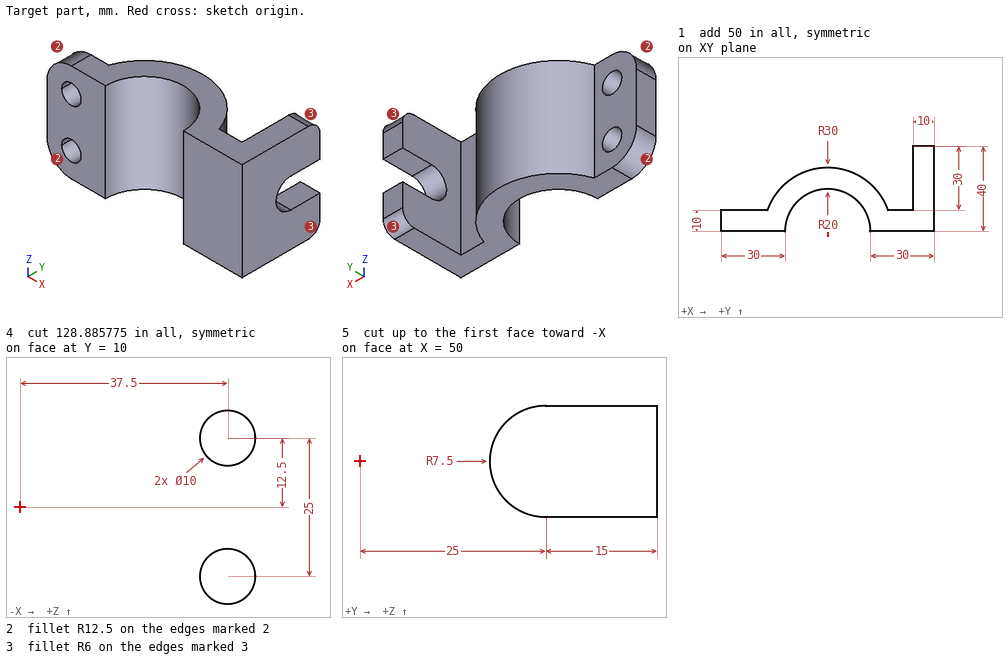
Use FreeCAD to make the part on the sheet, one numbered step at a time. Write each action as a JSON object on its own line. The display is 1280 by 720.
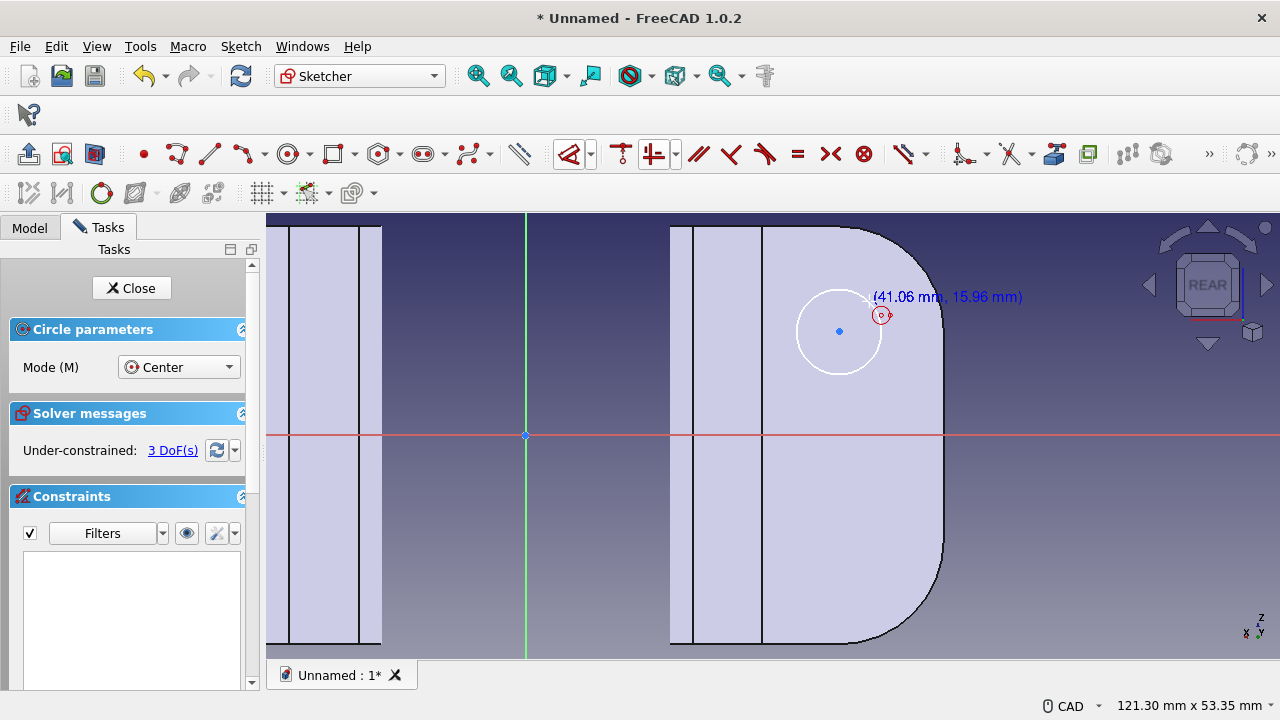
{"action": "left_click", "coordinate": [839, 540]}
{"action": "left_click", "coordinate": [869, 510]}
{"action": "key", "text": "Escape"}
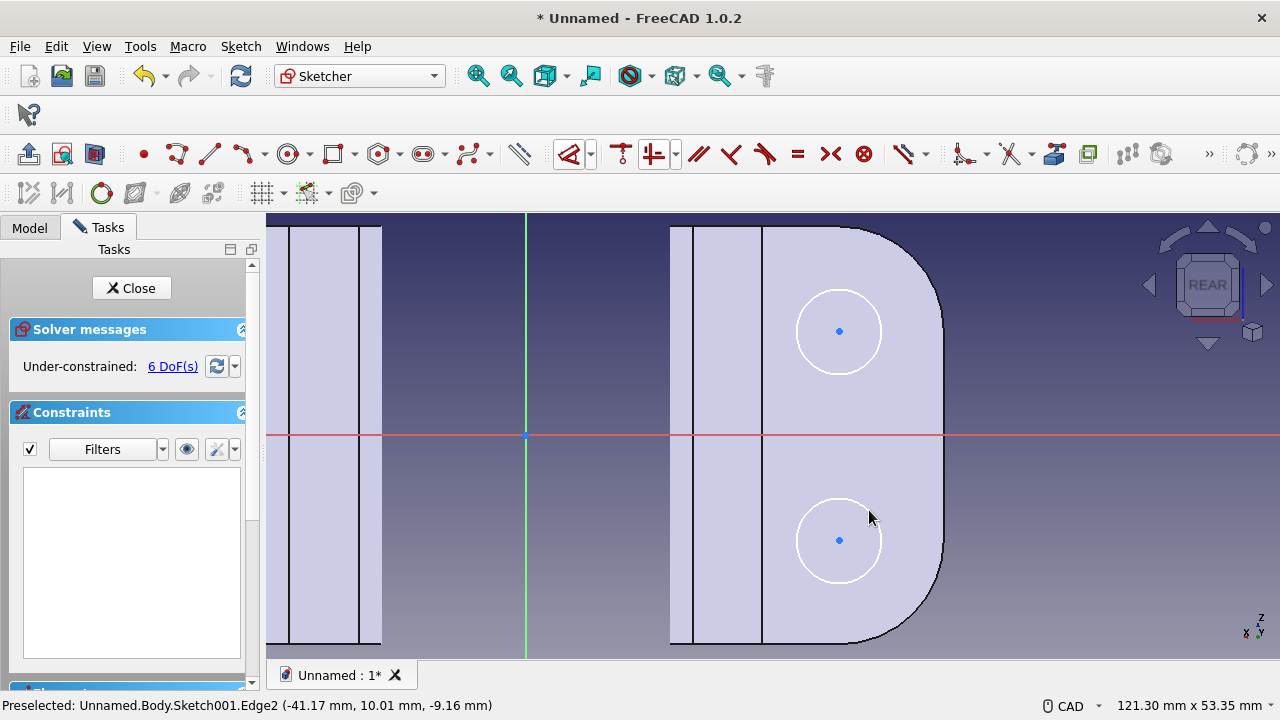
{"action": "left_click", "coordinate": [869, 302]}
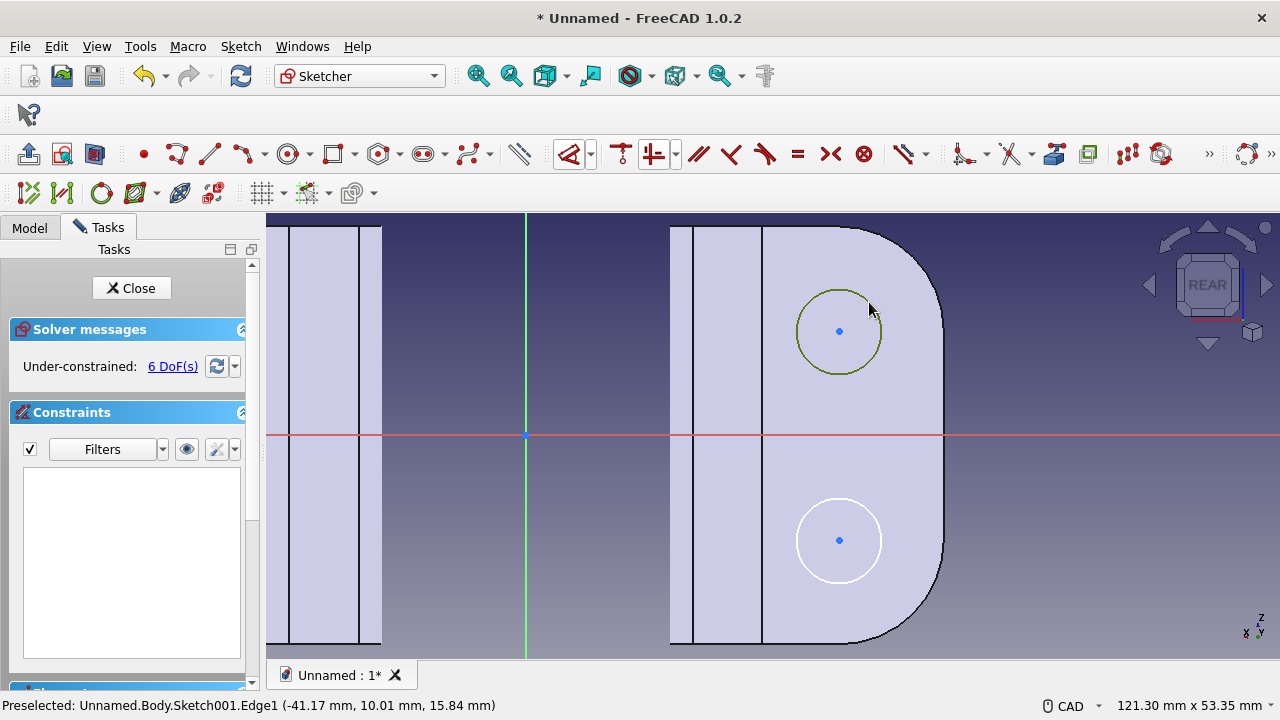
{"action": "left_click", "coordinate": [869, 511]}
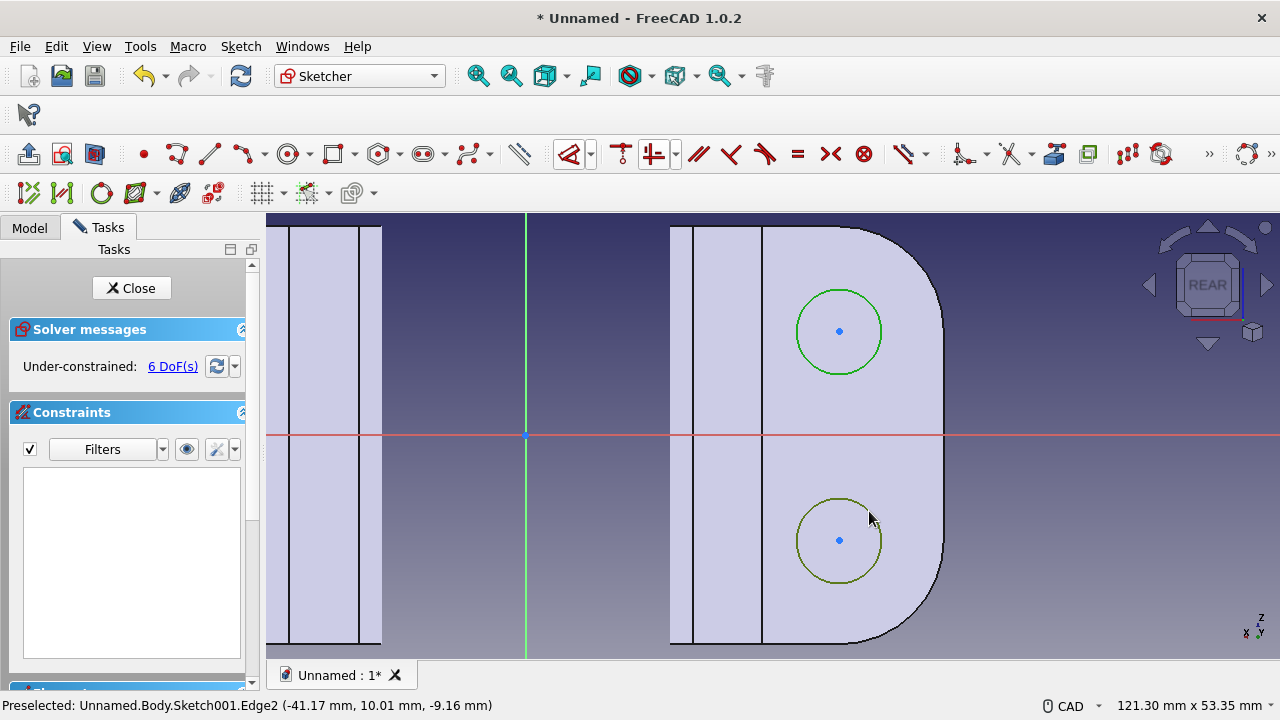
{"action": "left_click", "coordinate": [798, 154]}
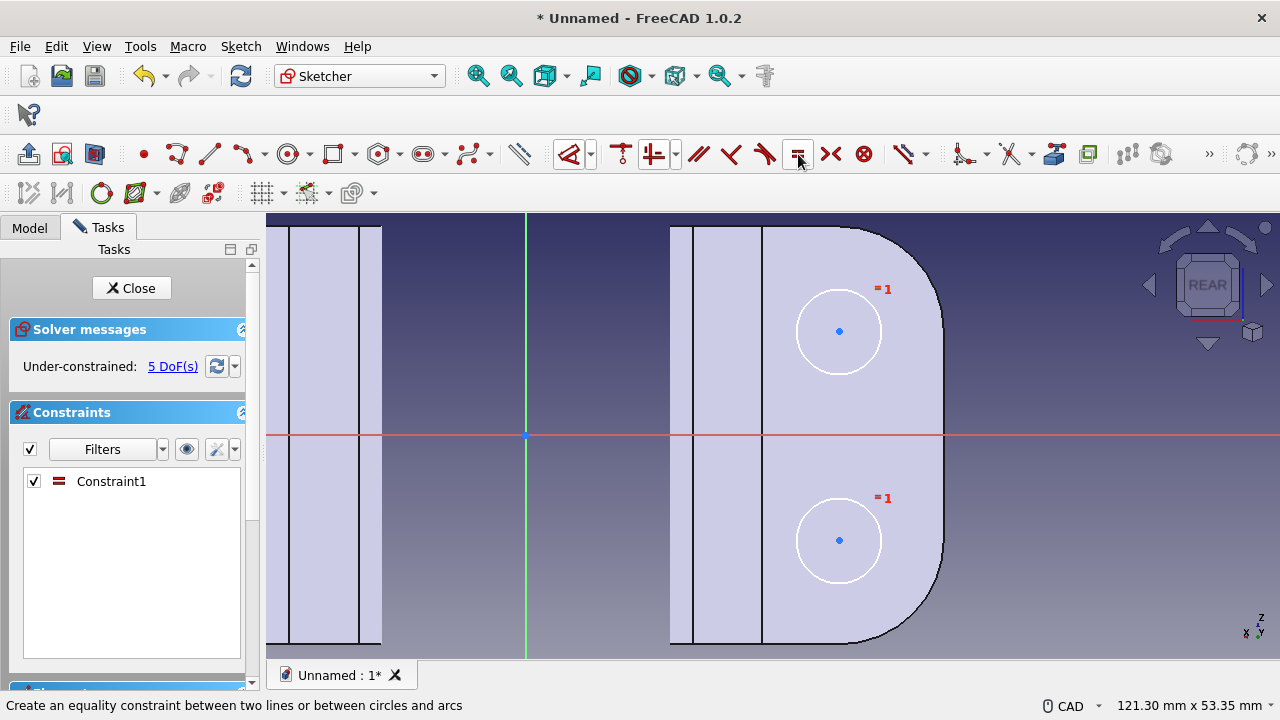
{"action": "left_click", "coordinate": [839, 332]}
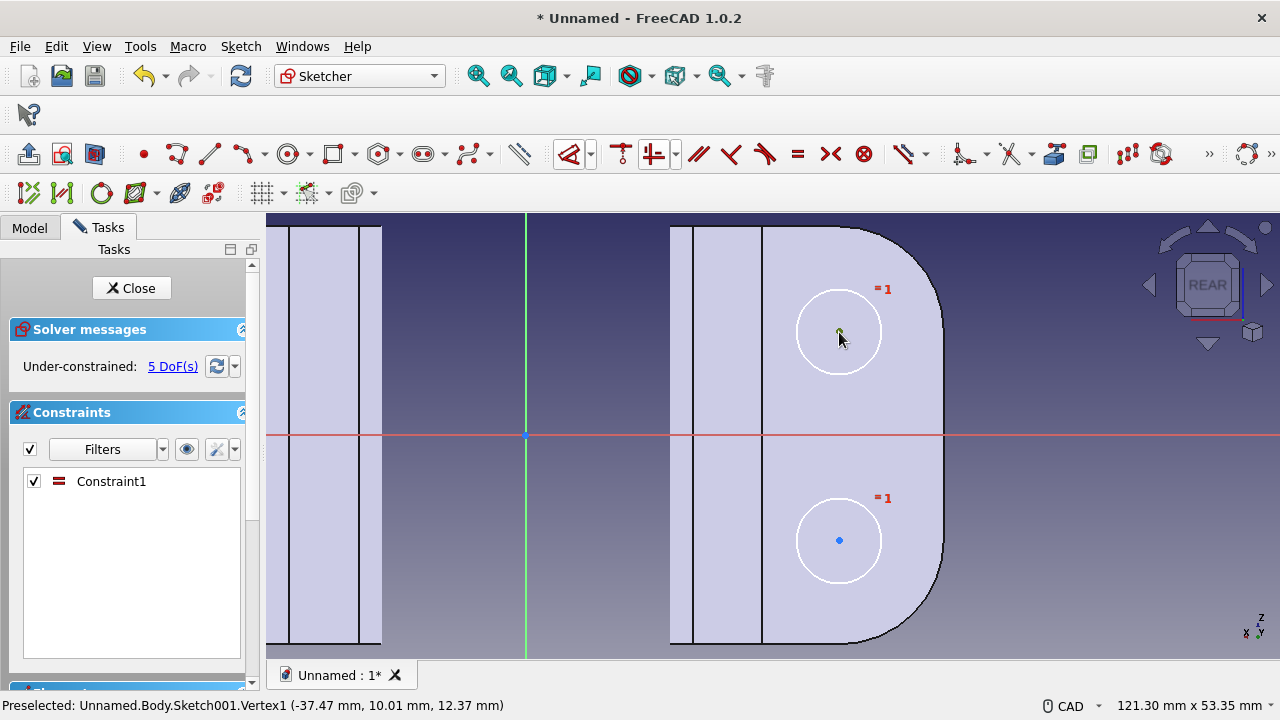
{"action": "left_click", "coordinate": [839, 541]}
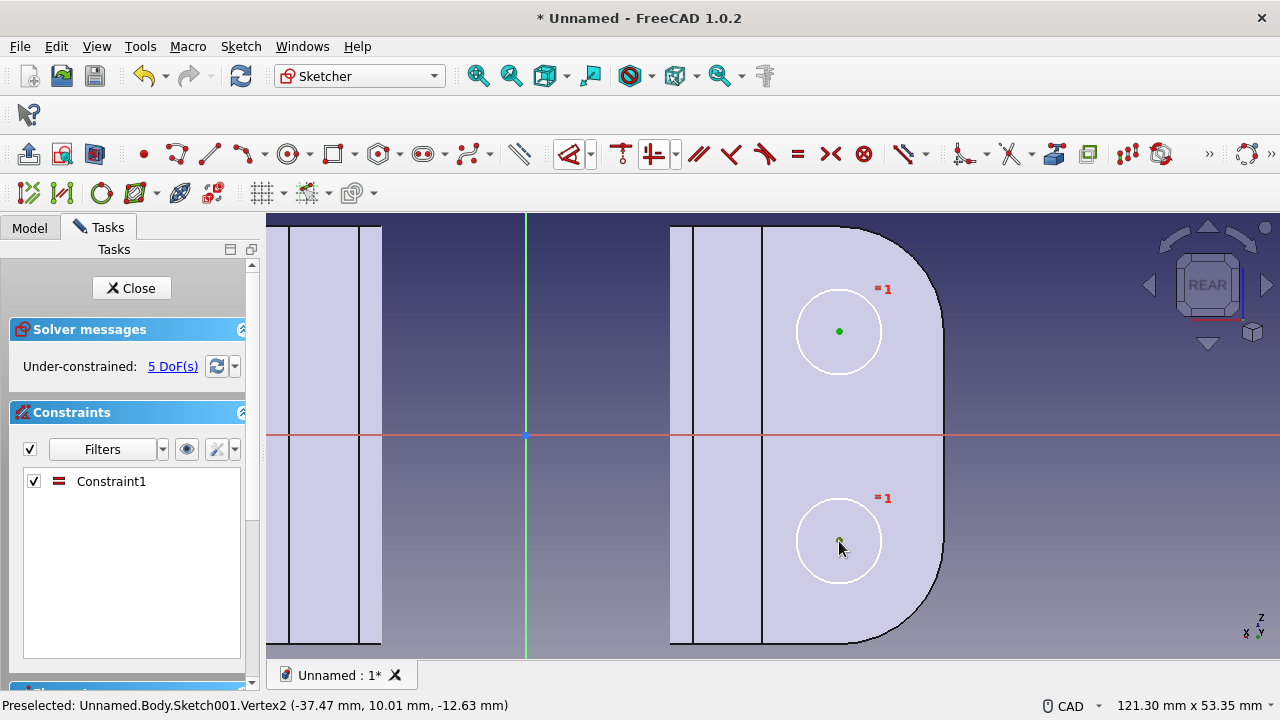
{"action": "left_click", "coordinate": [676, 154]}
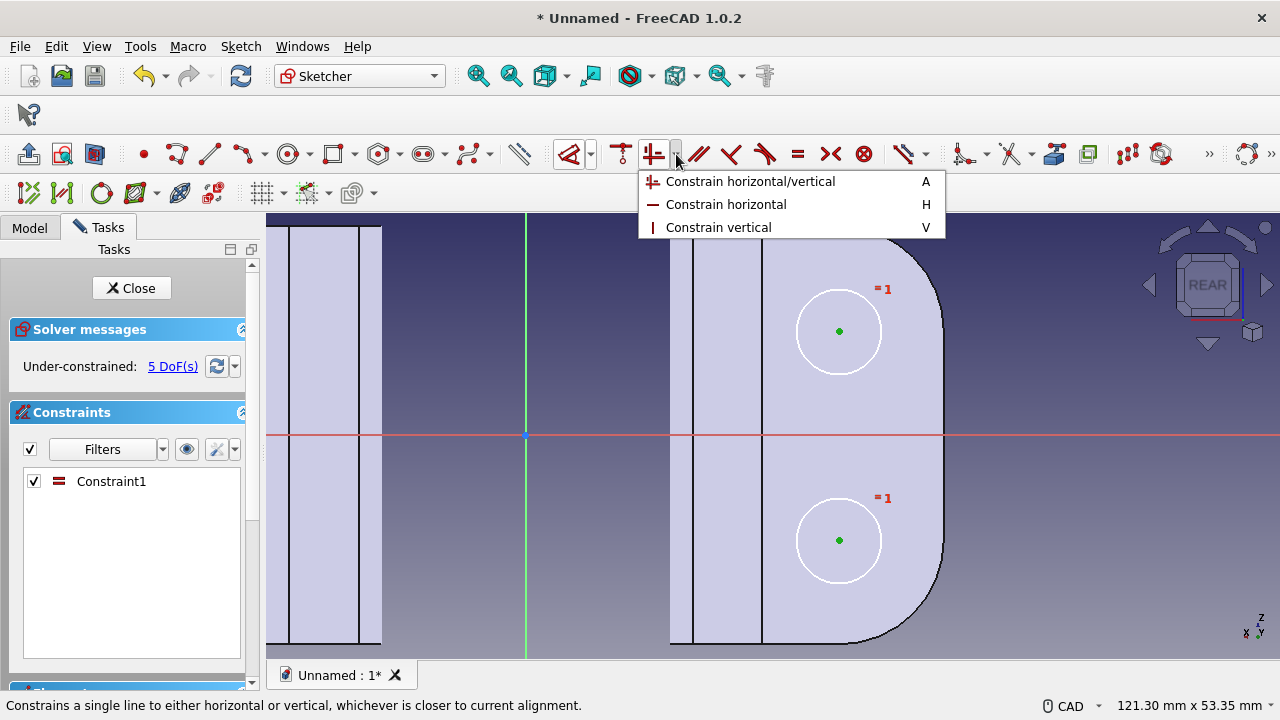
{"action": "left_click", "coordinate": [792, 228]}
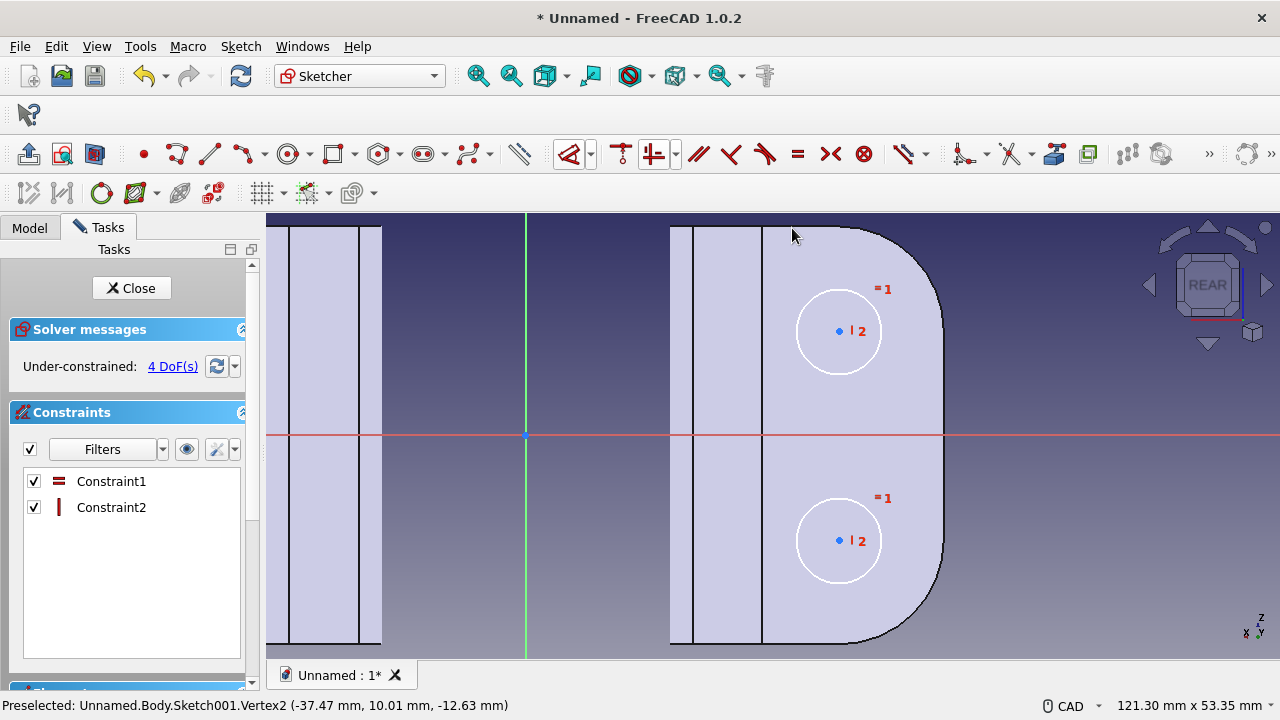
{"action": "left_click", "coordinate": [869, 302]}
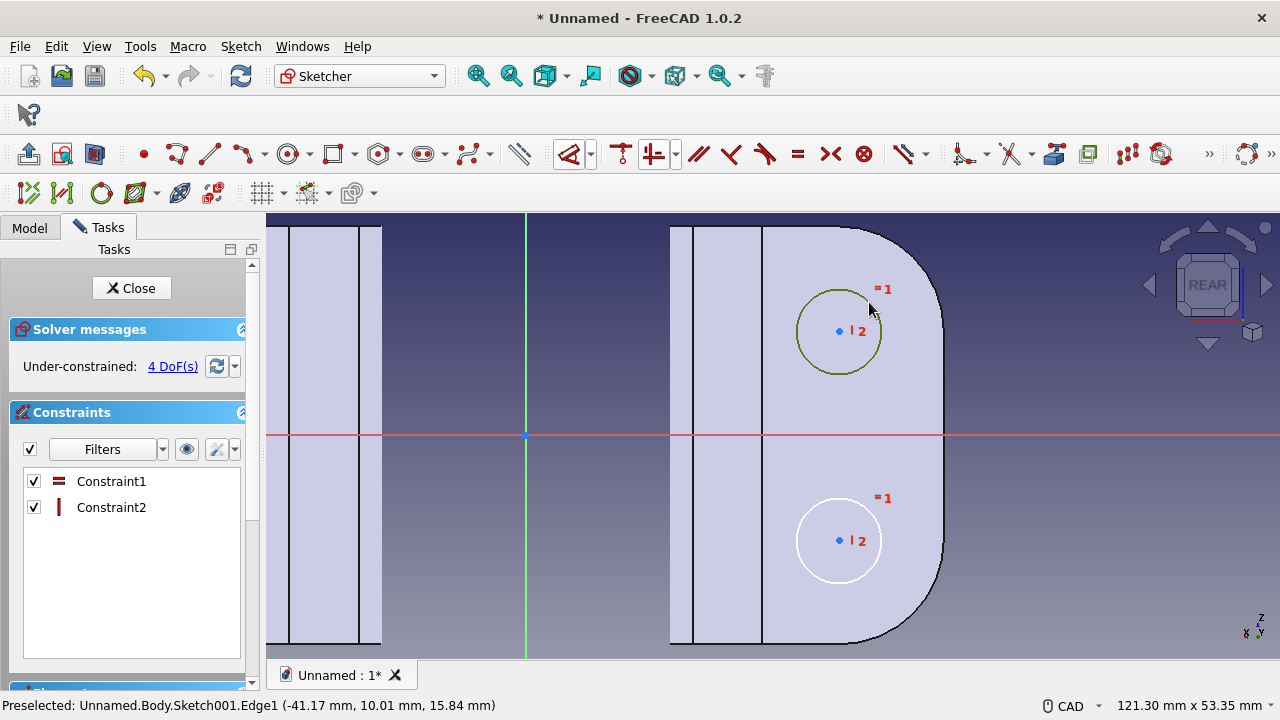
{"action": "left_click", "coordinate": [590, 154]}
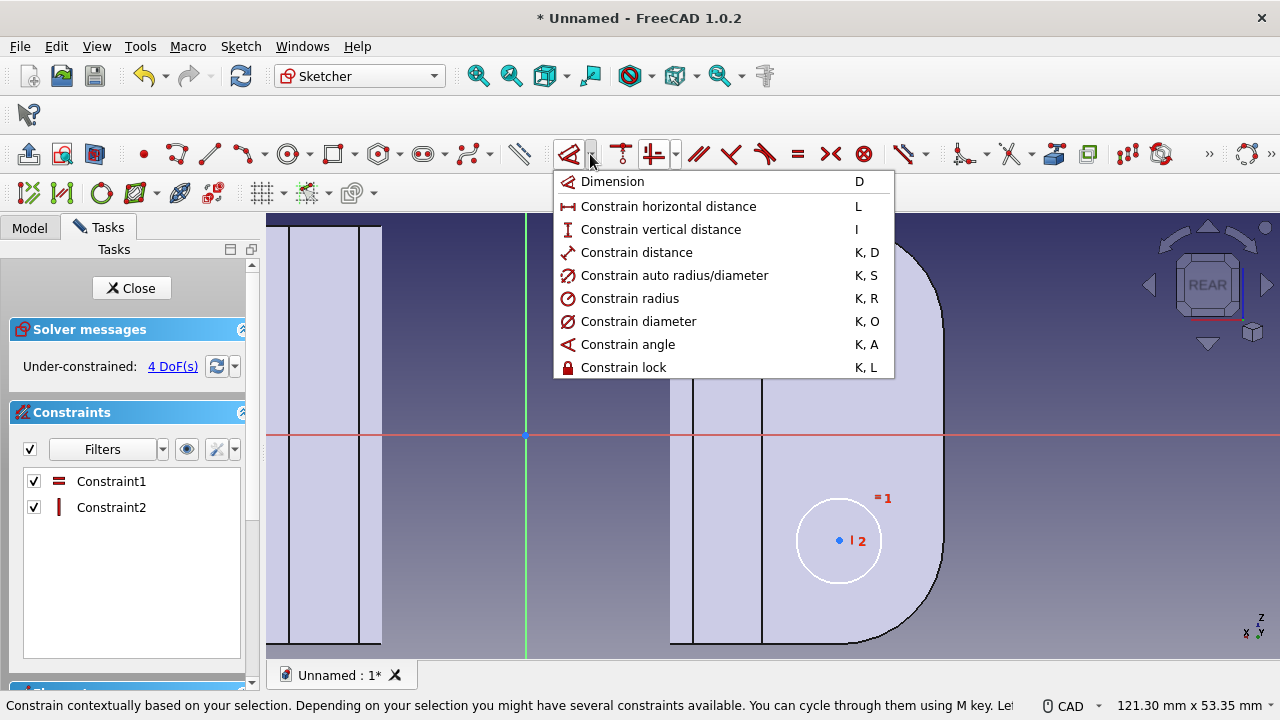
{"action": "left_click", "coordinate": [724, 322]}